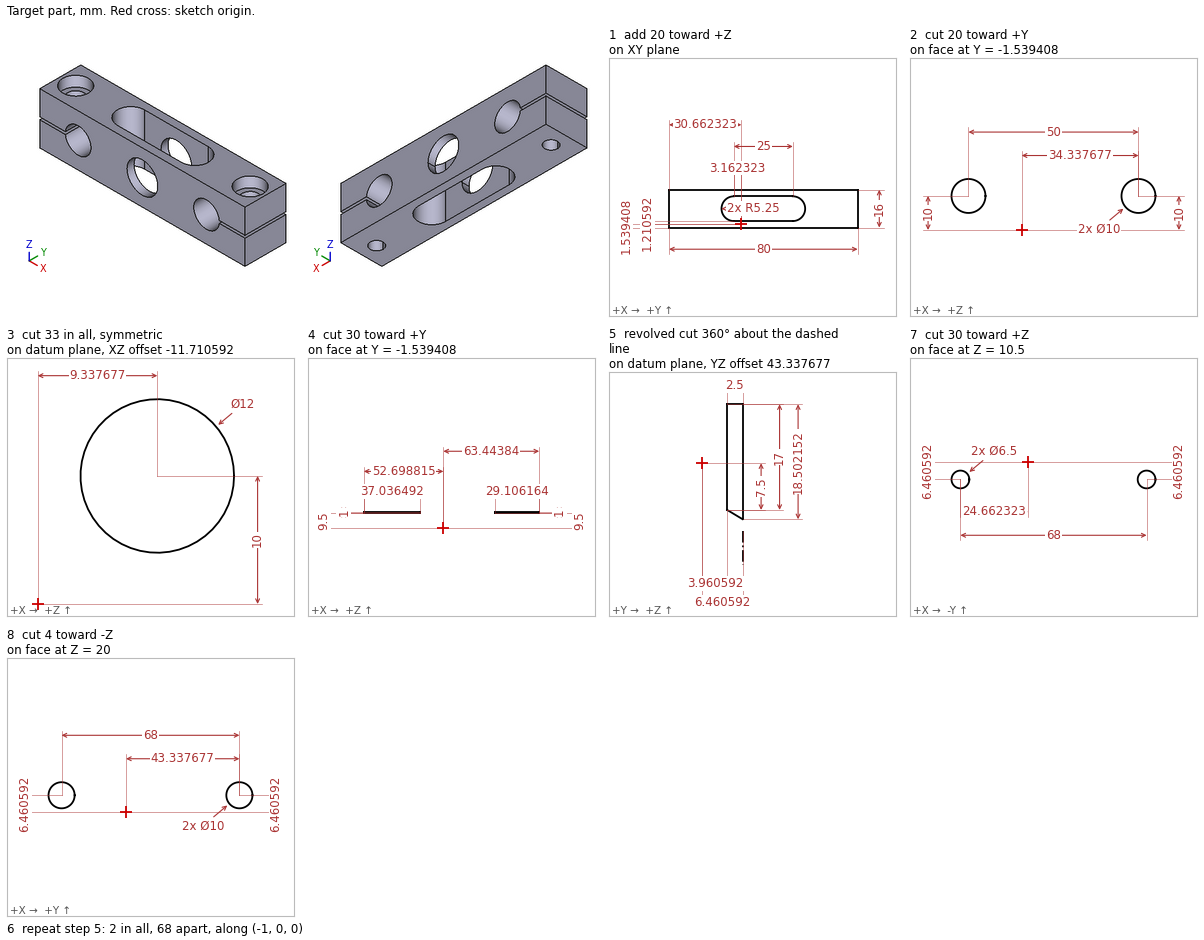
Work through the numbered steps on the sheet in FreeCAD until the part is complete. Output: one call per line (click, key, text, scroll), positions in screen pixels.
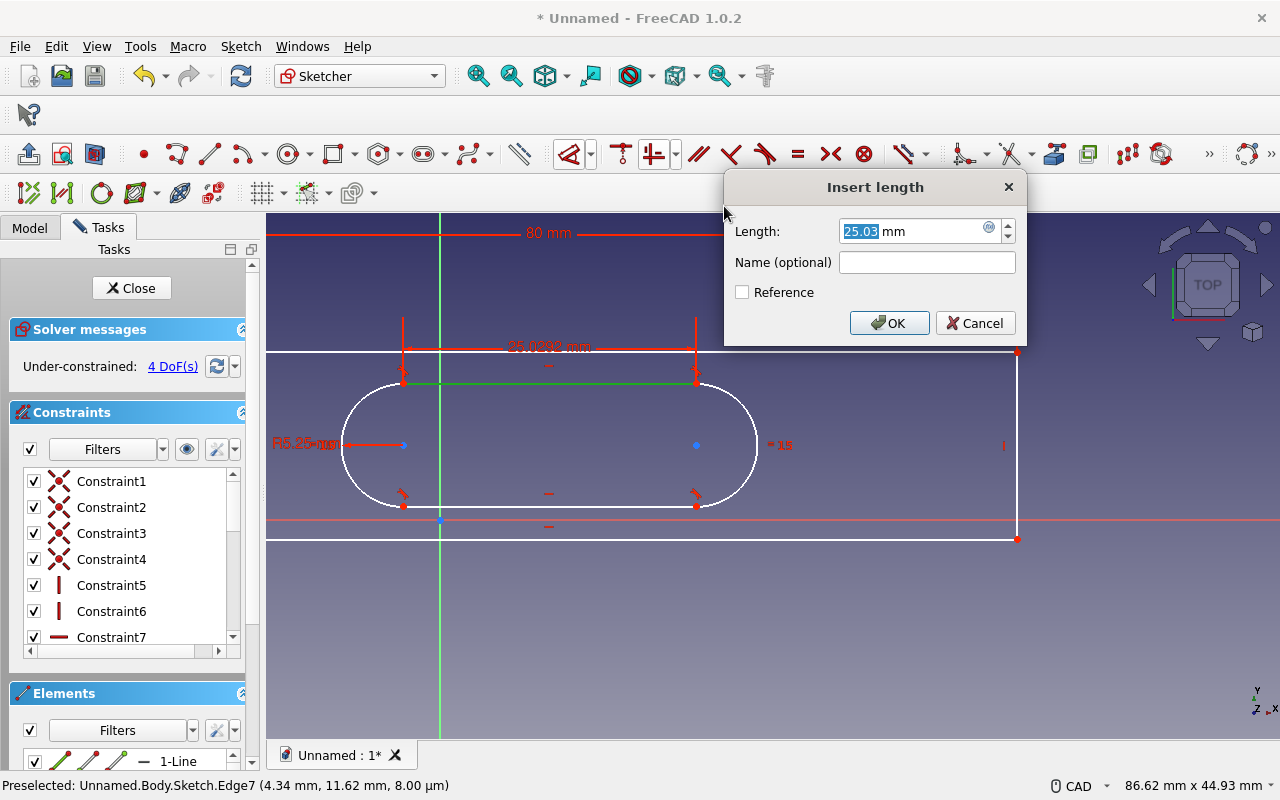
text(25)
key(Return)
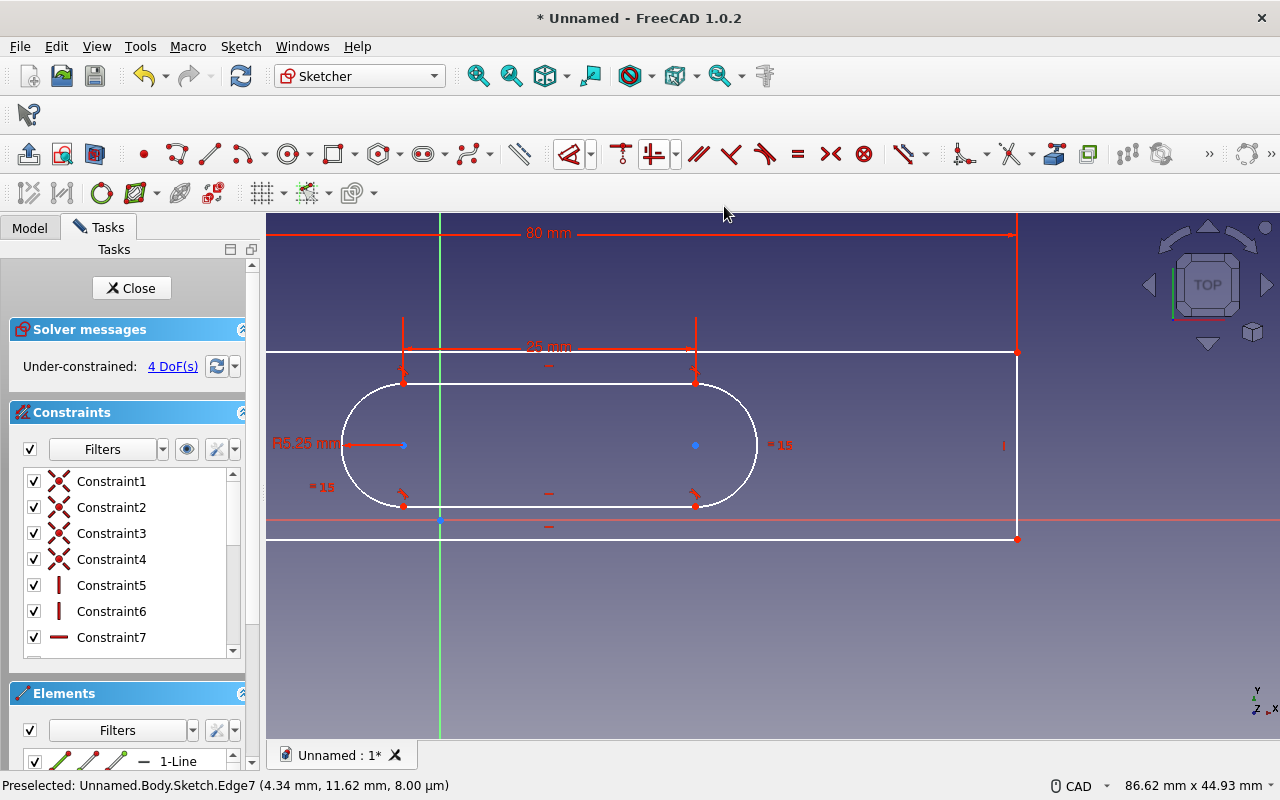
scroll(1020, 540, down, 2)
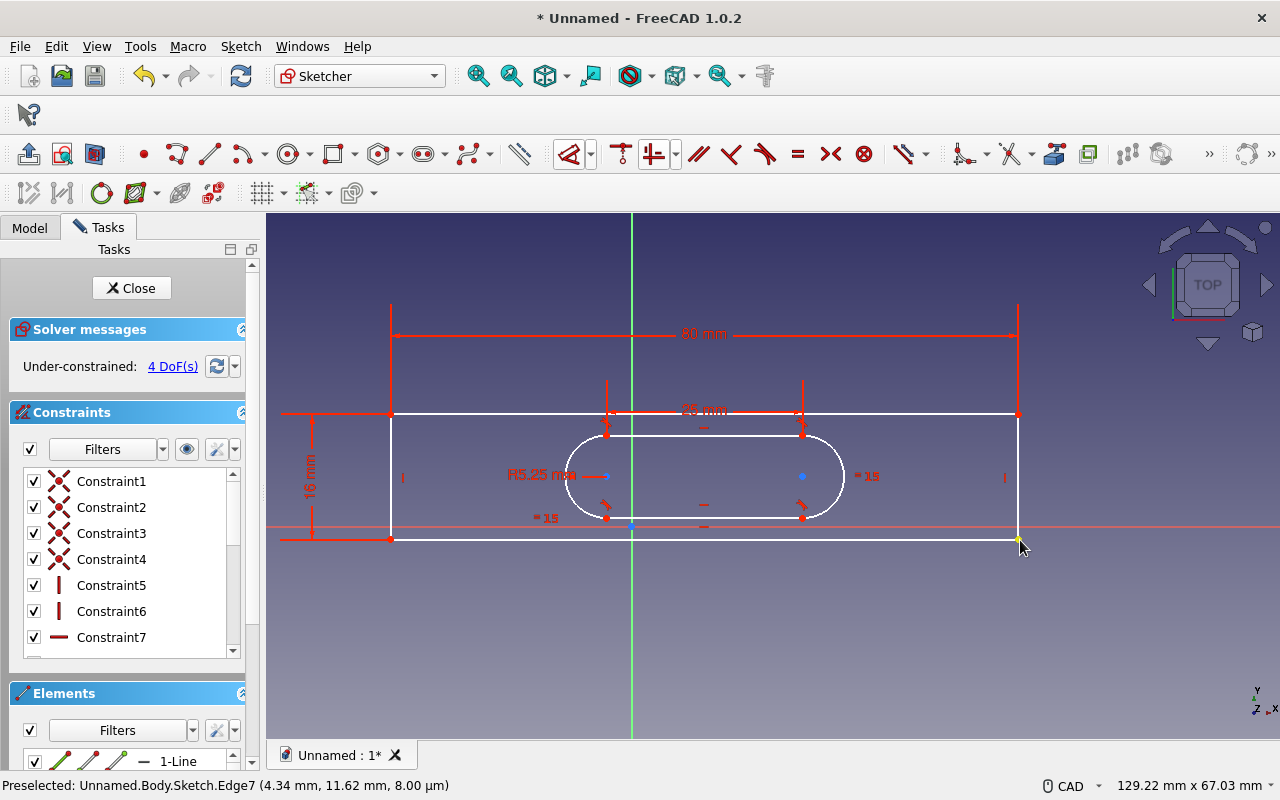
scroll(391, 540, up, 6)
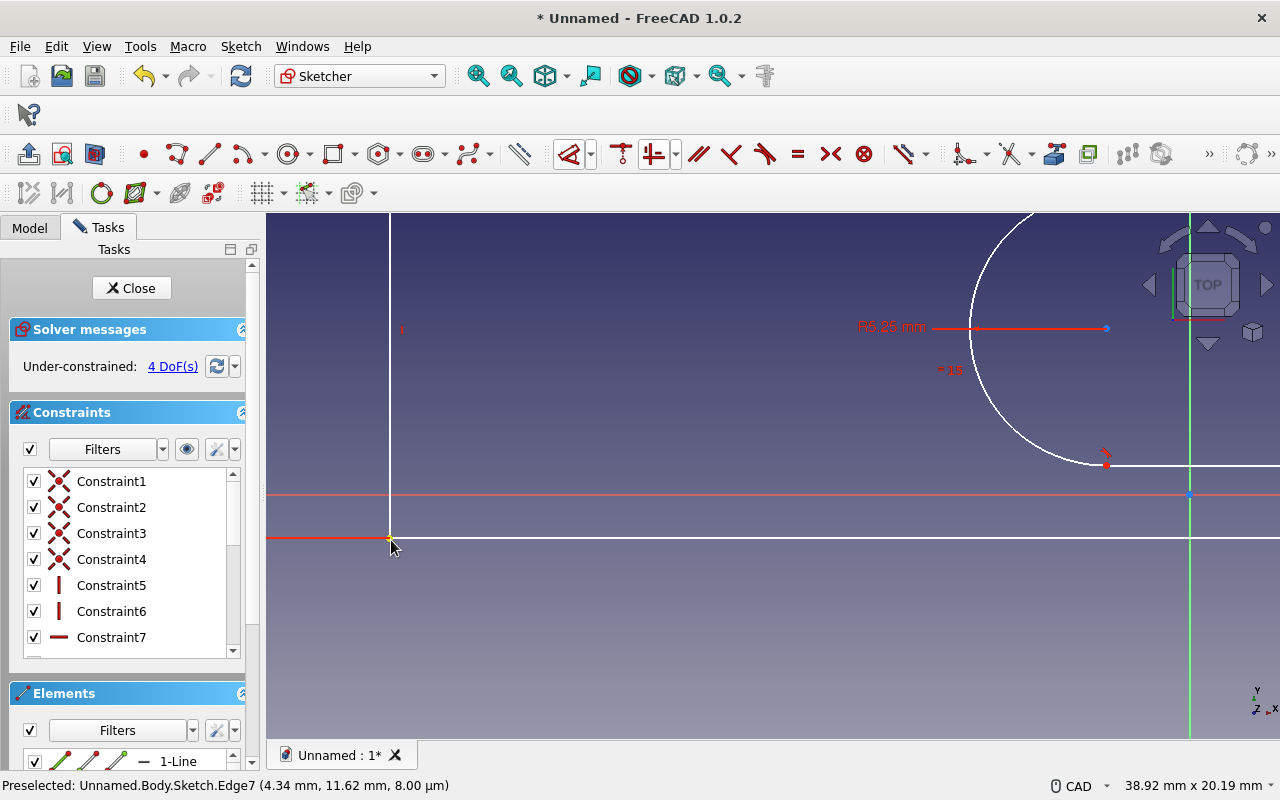
click(390, 538)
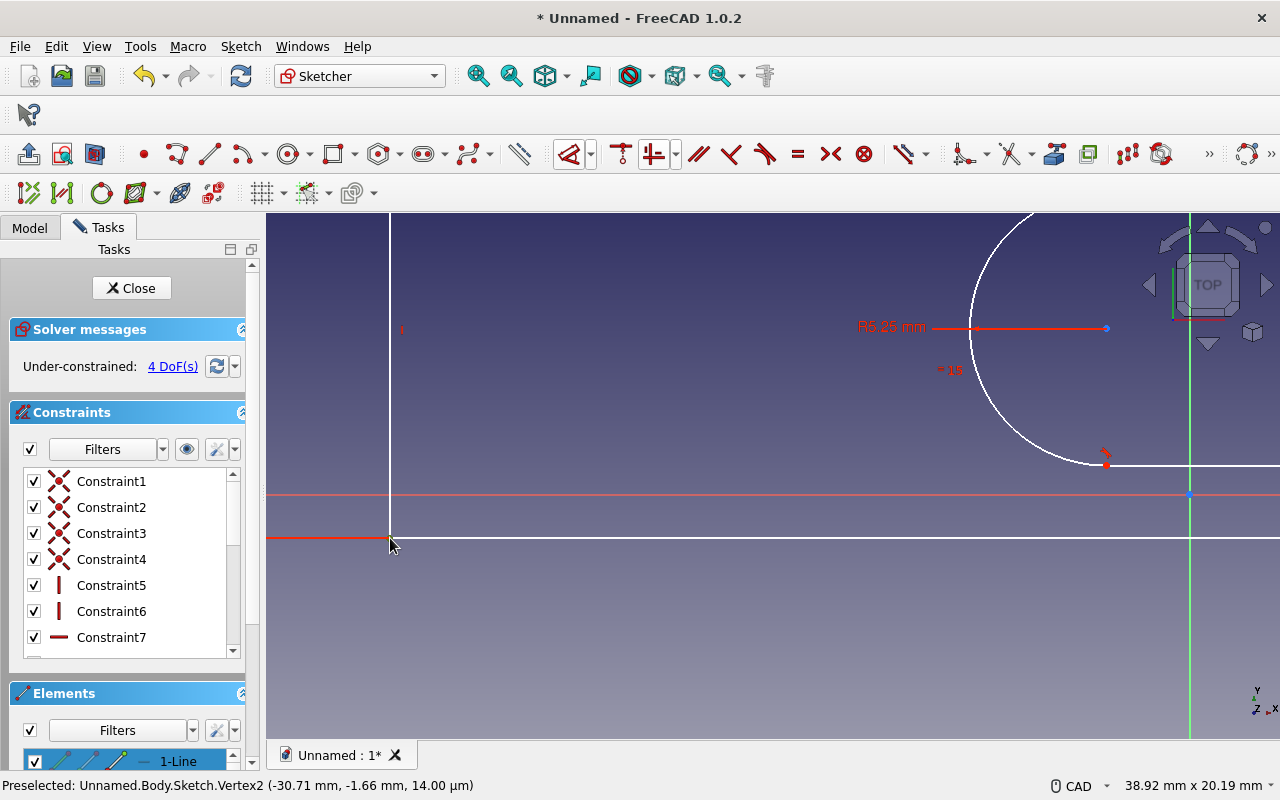
click(590, 154)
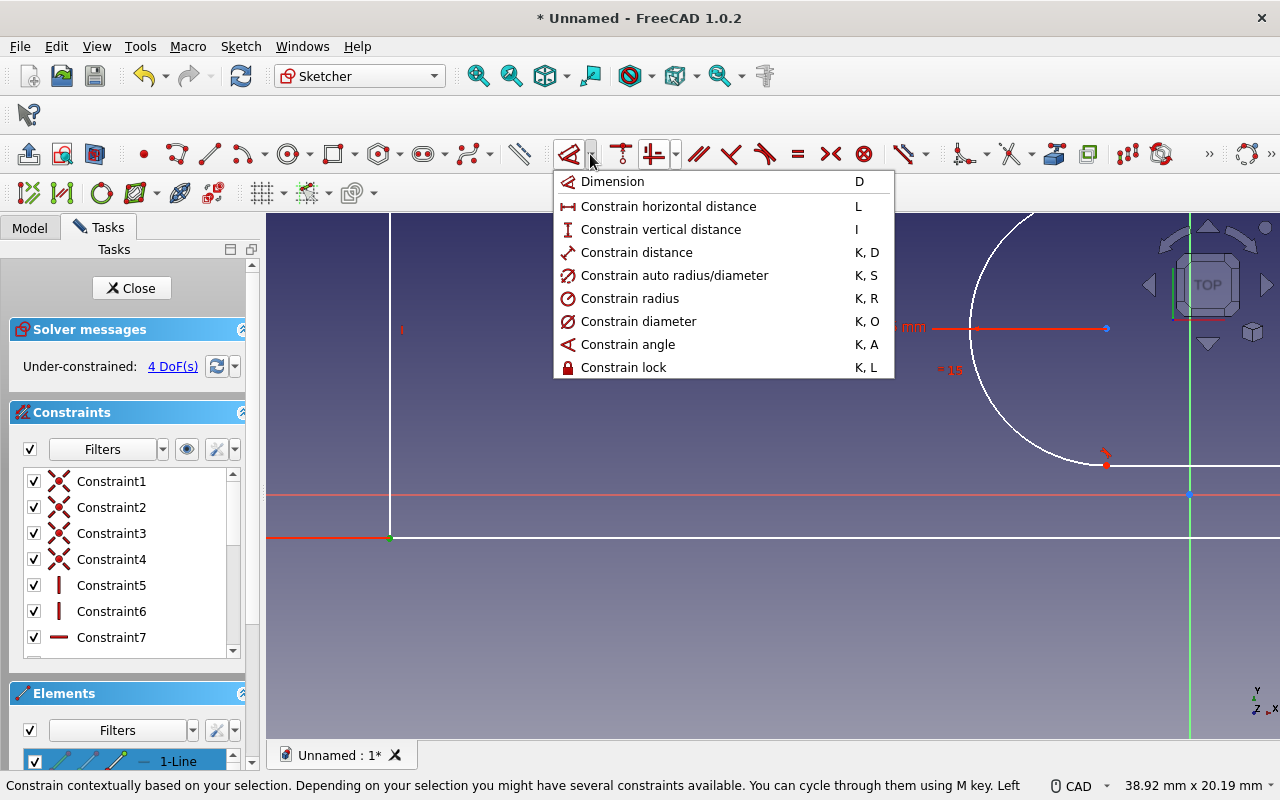
click(724, 230)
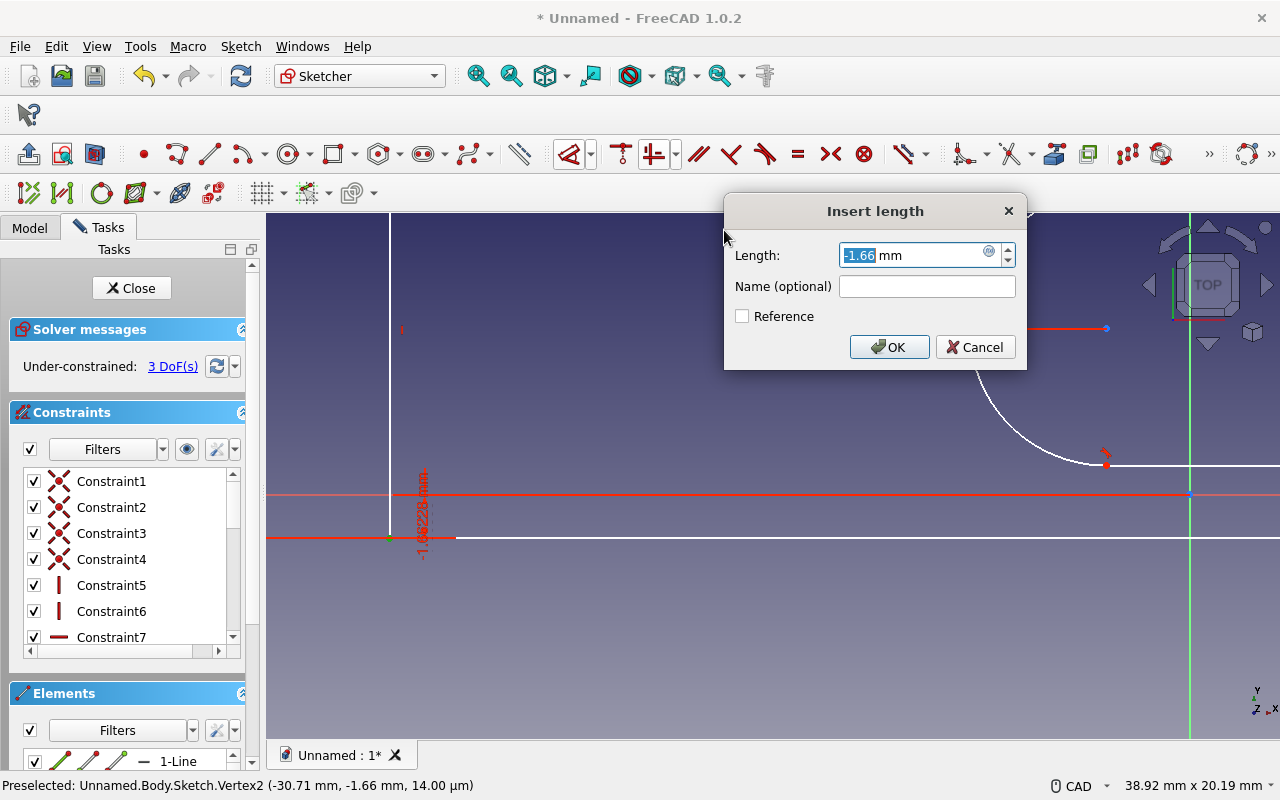
text(-1.539408)
key(Return)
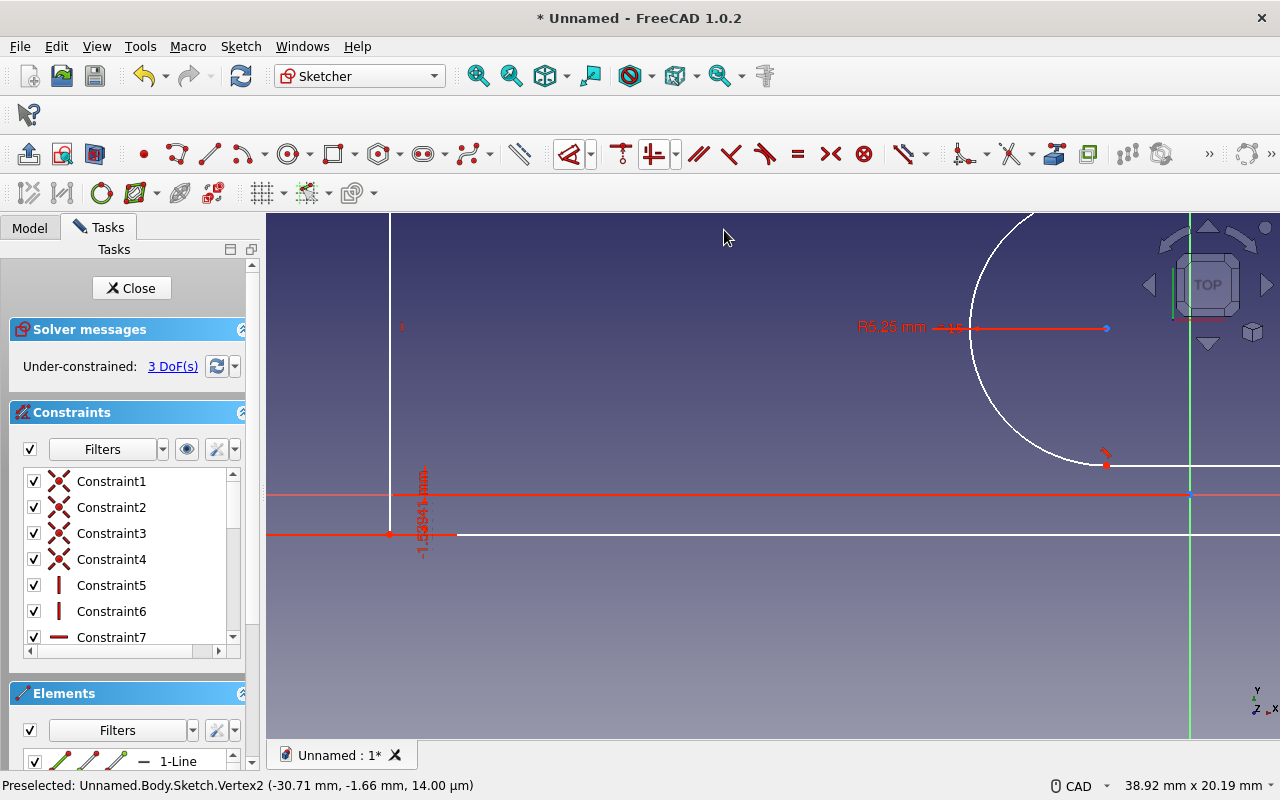
scroll(391, 540, down, 6)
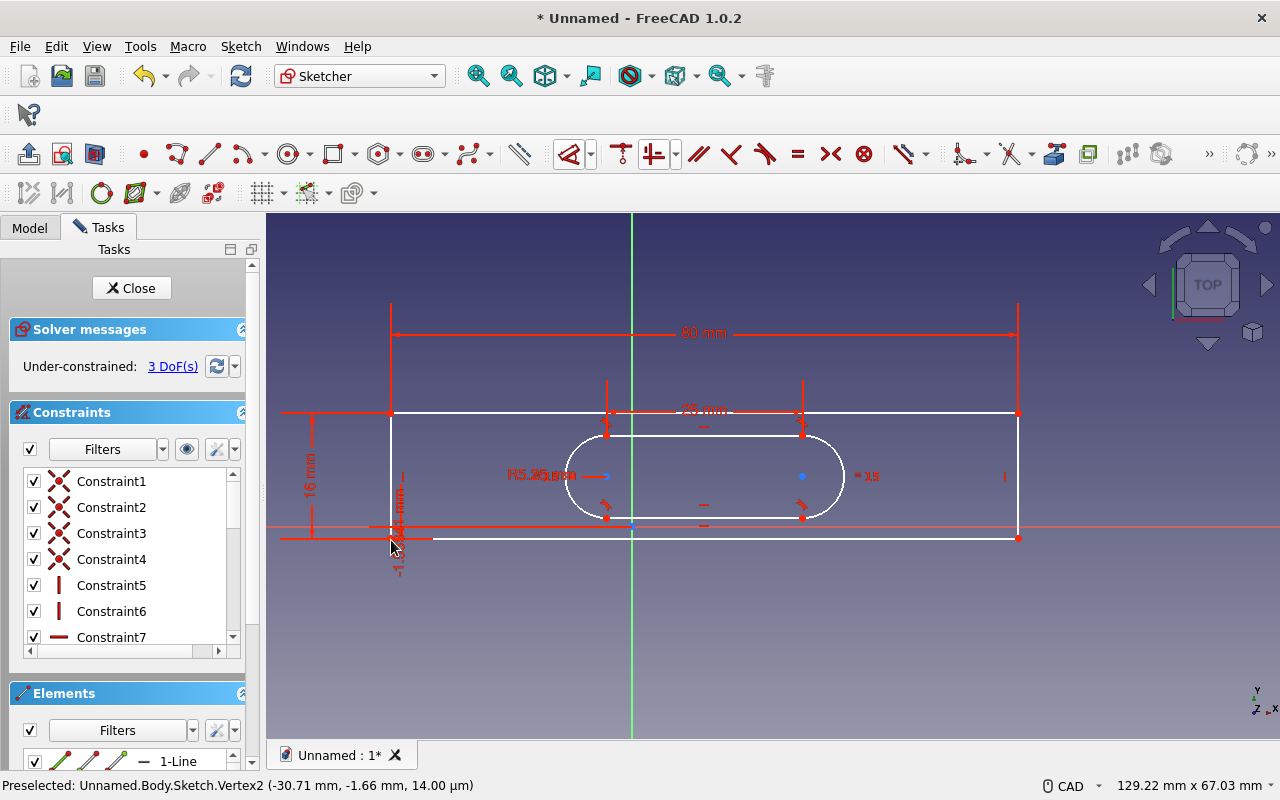
scroll(607, 436, up, 3)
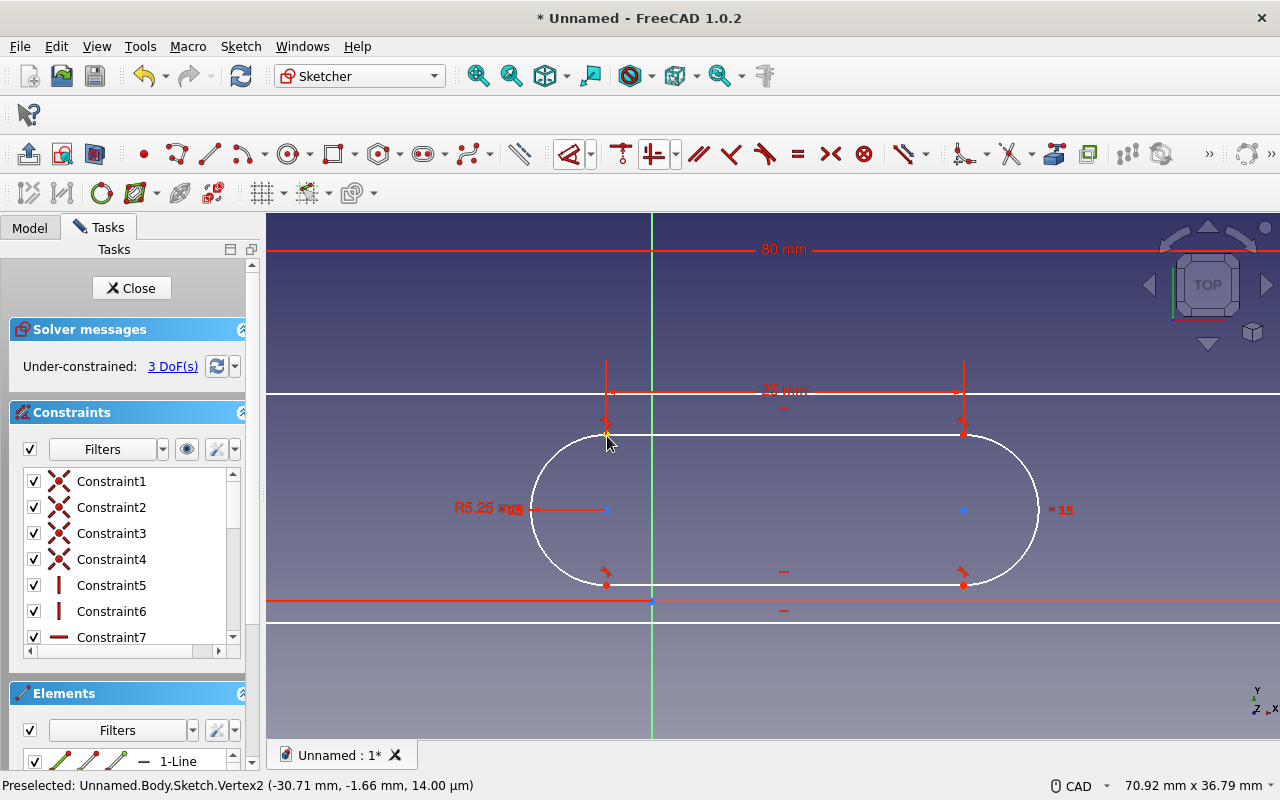
click(606, 435)